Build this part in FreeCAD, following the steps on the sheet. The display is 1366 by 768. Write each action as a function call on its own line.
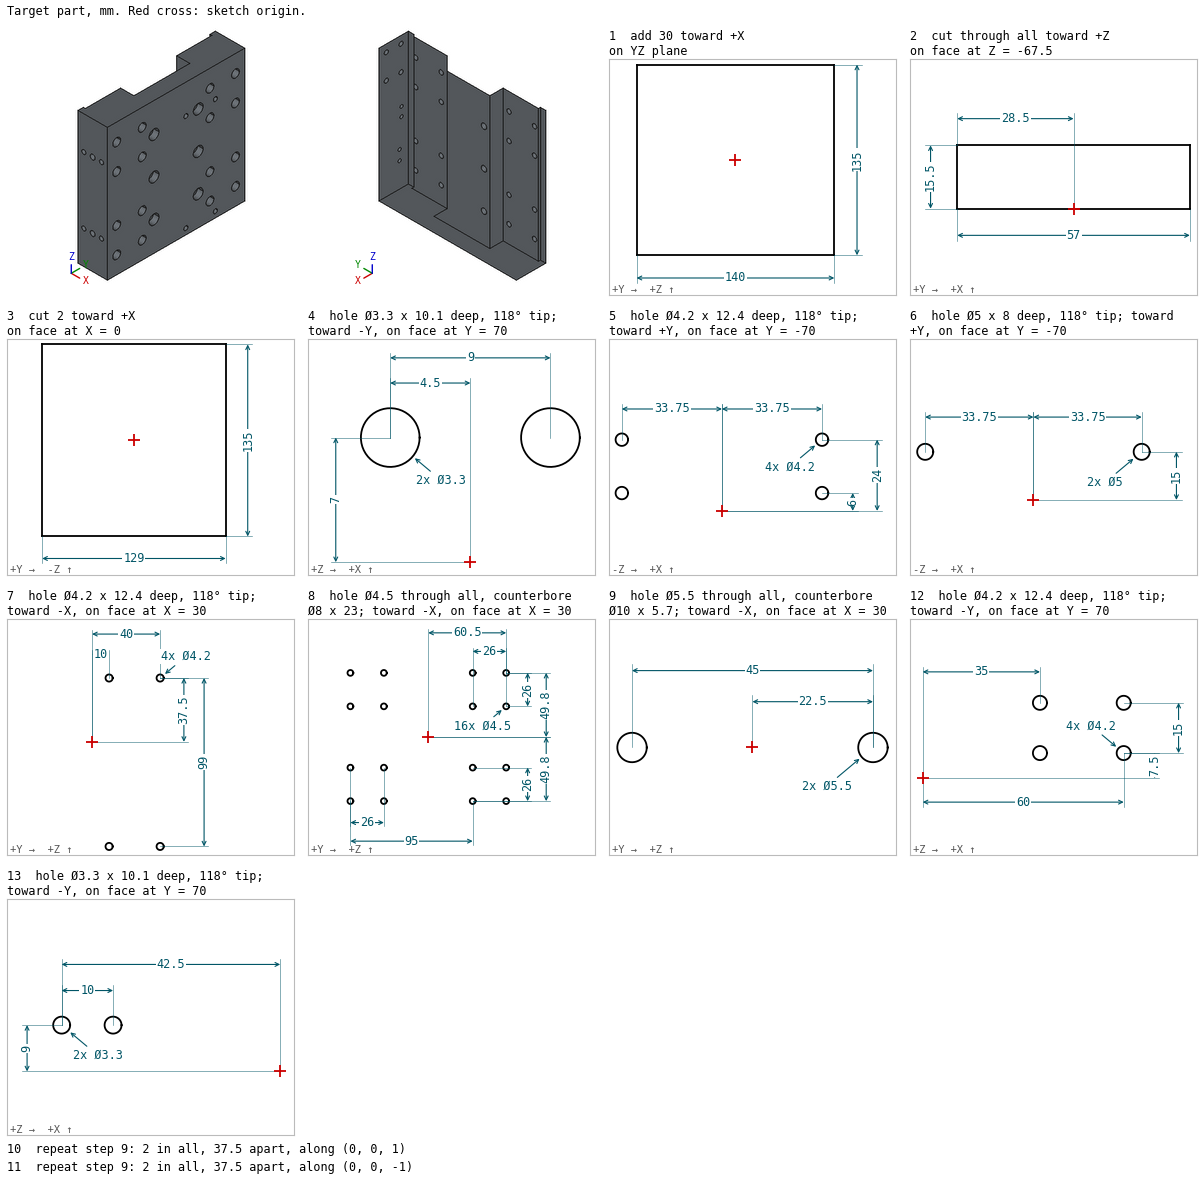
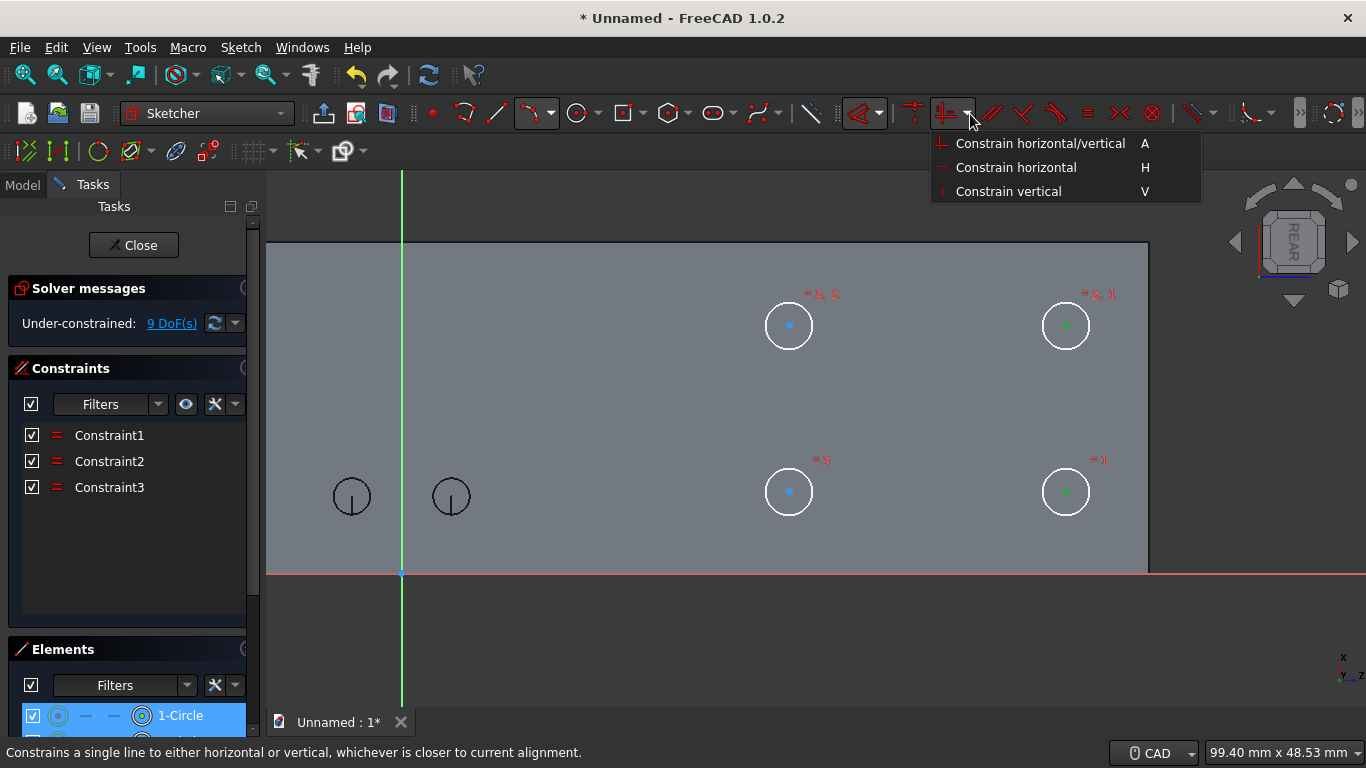
click(1066, 191)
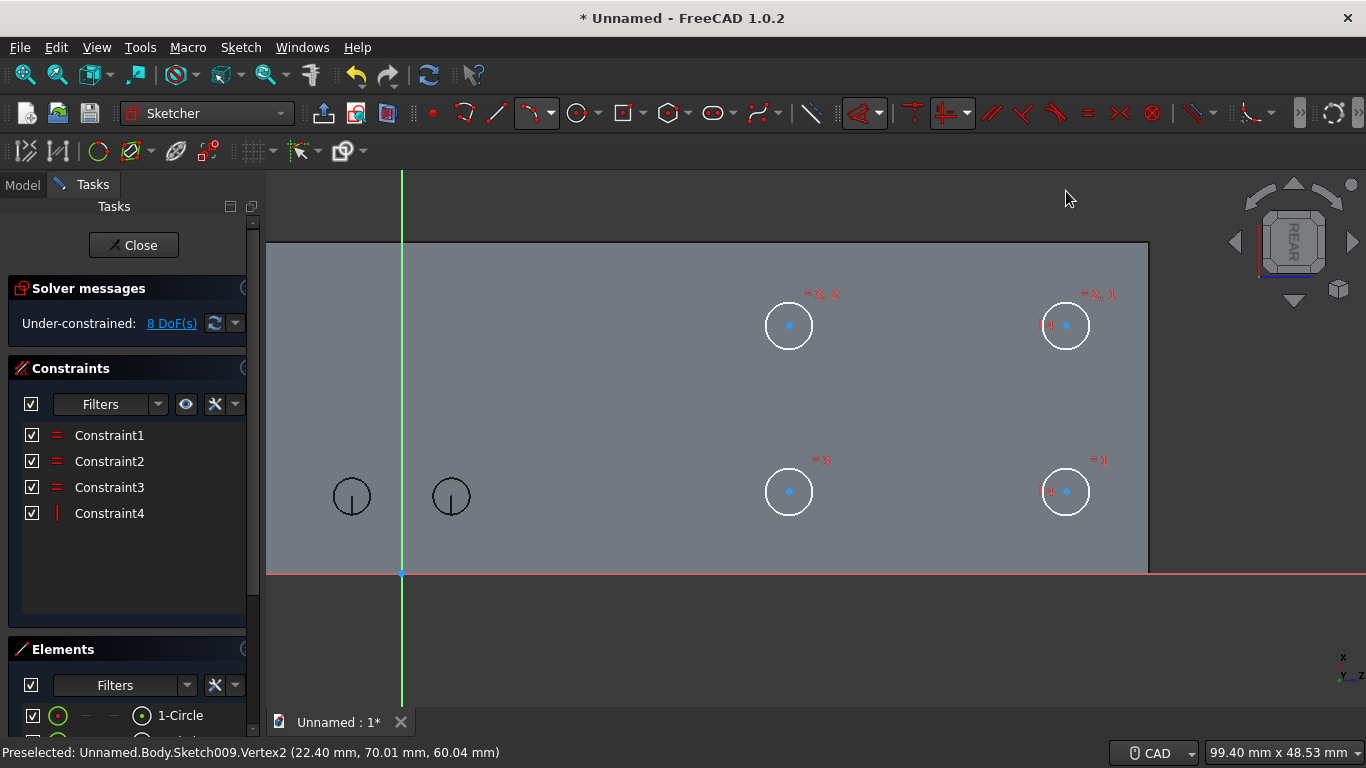
click(1066, 326)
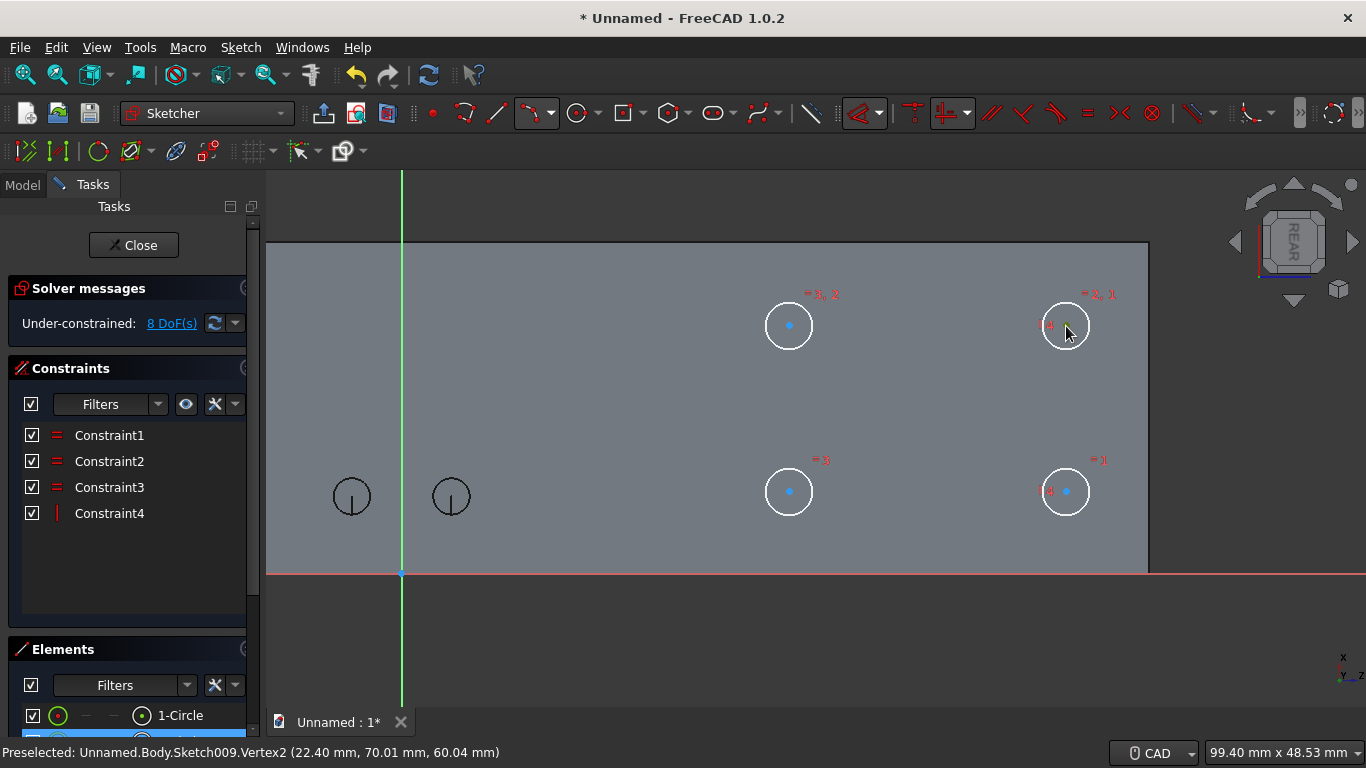
click(789, 326)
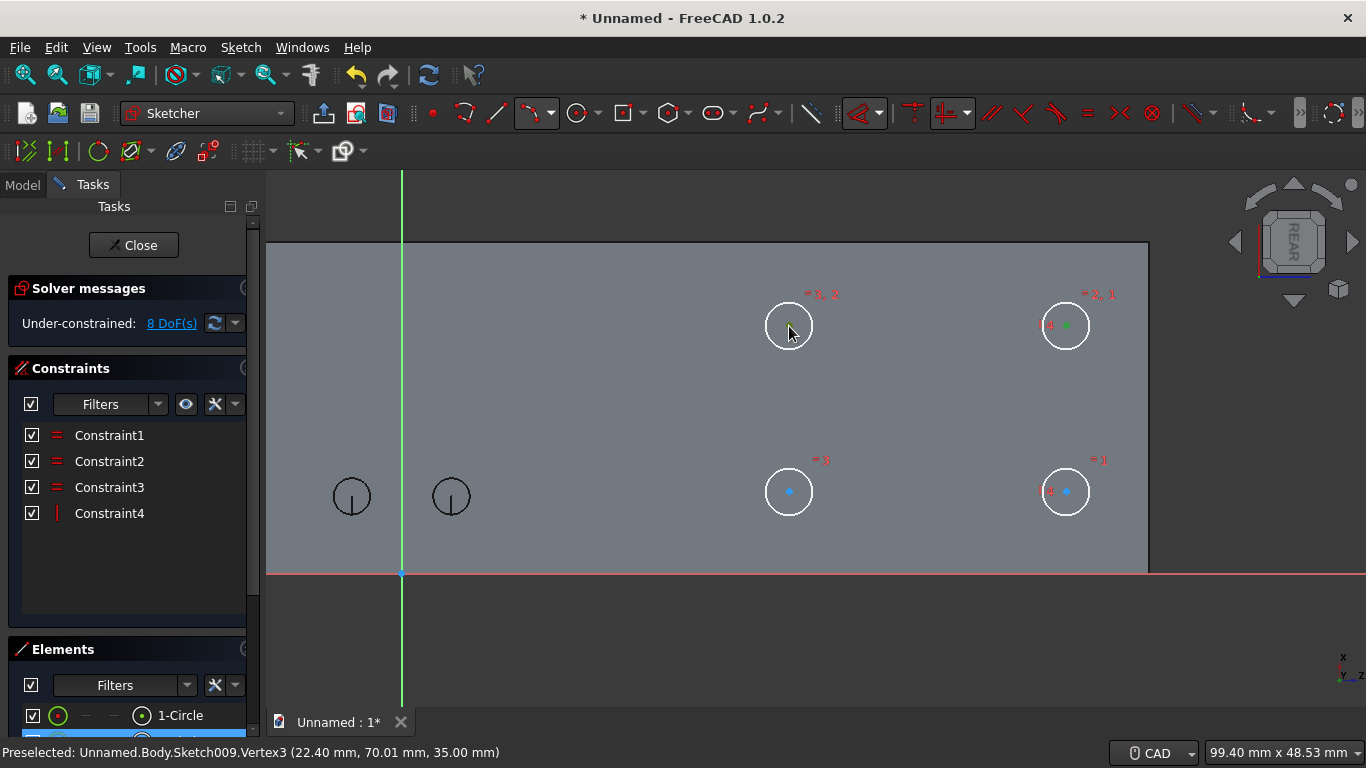
key(h)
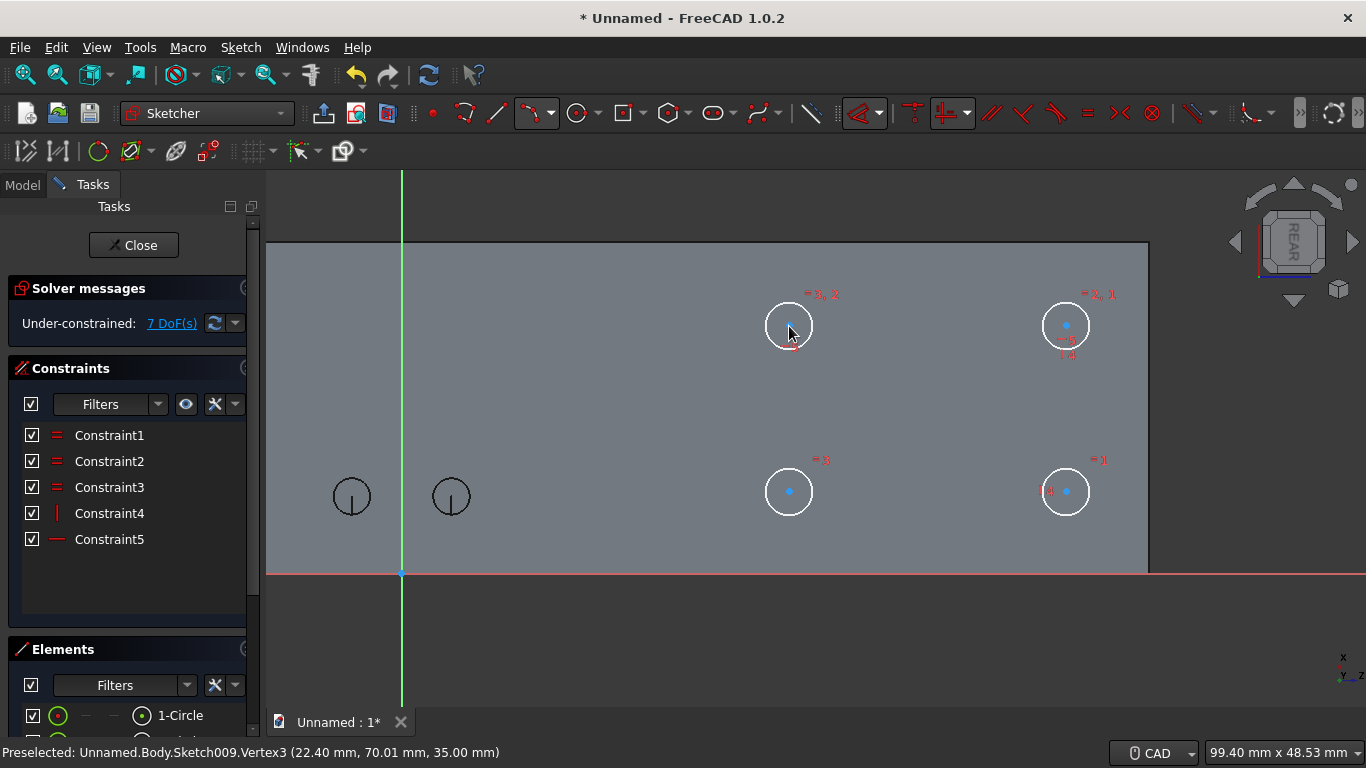
click(789, 326)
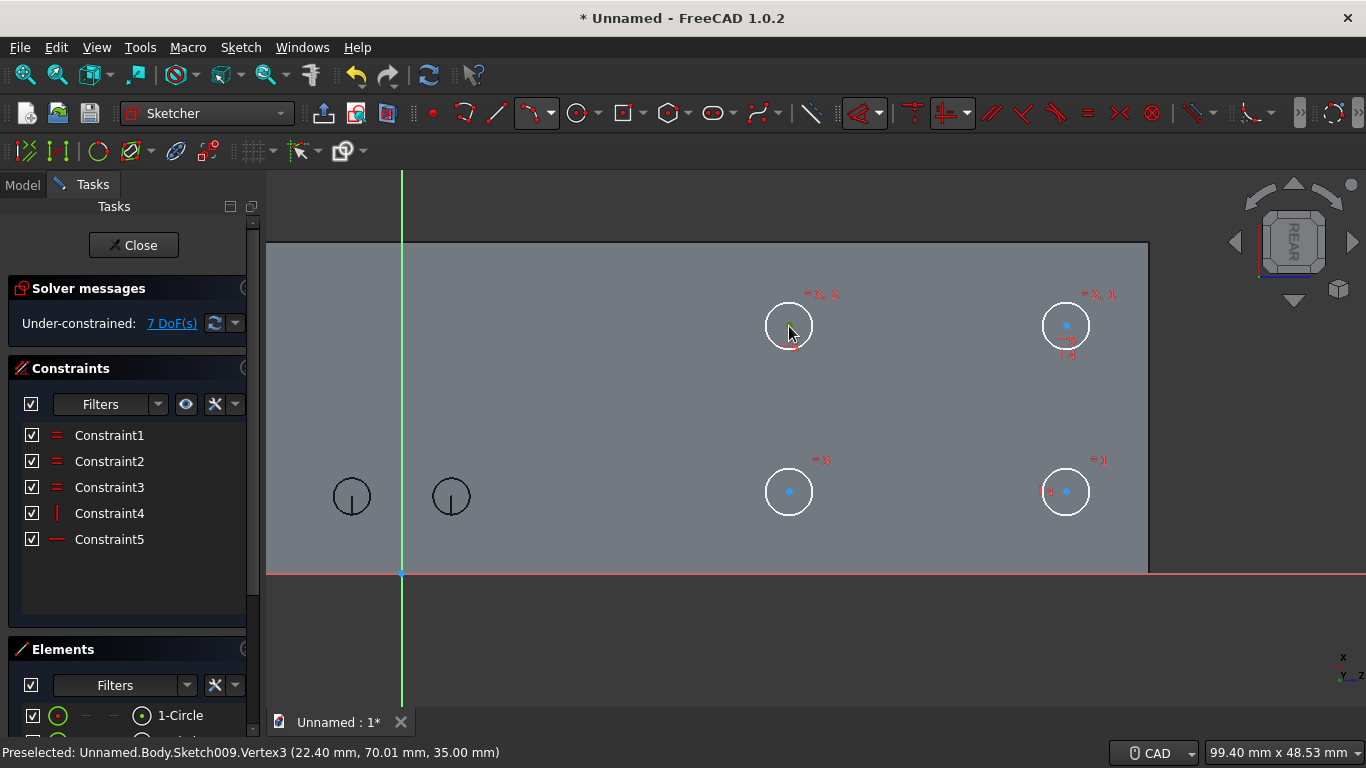
click(789, 492)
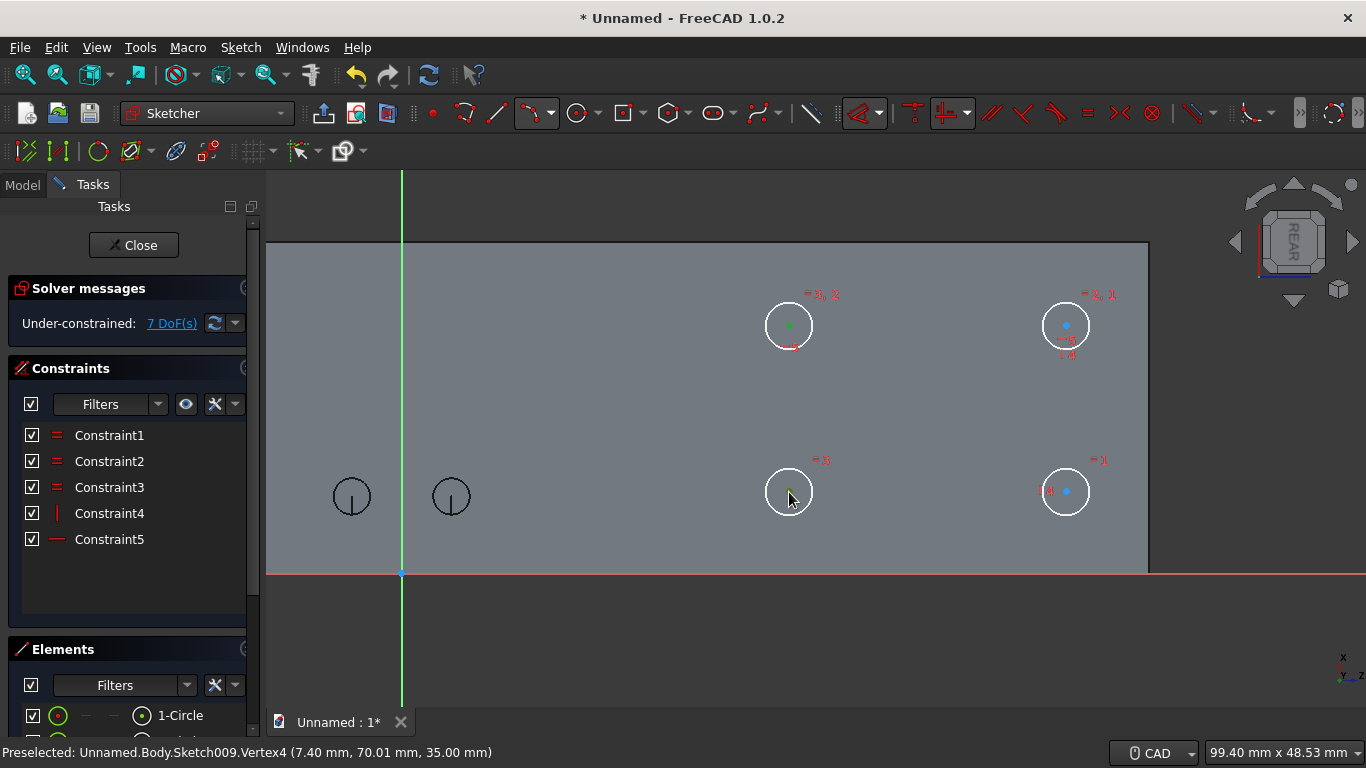
key(v)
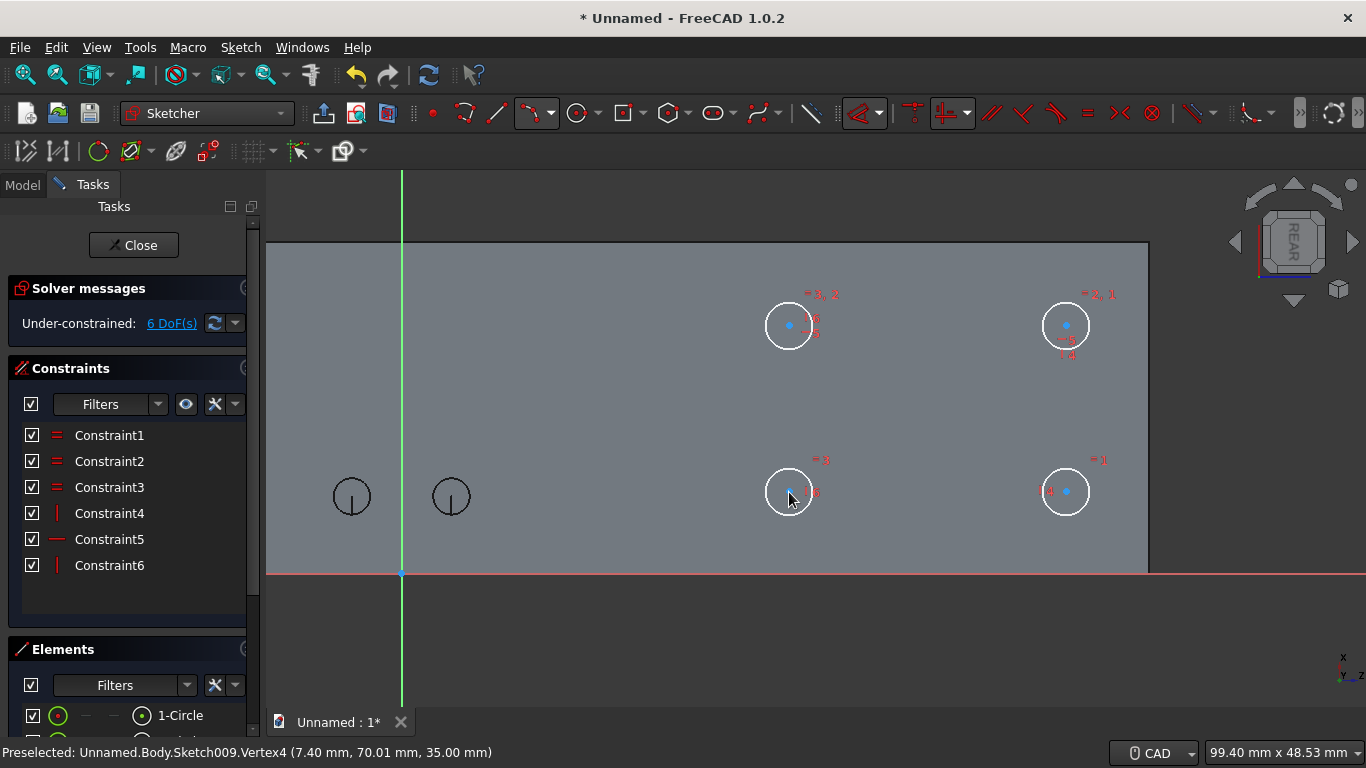
click(1066, 492)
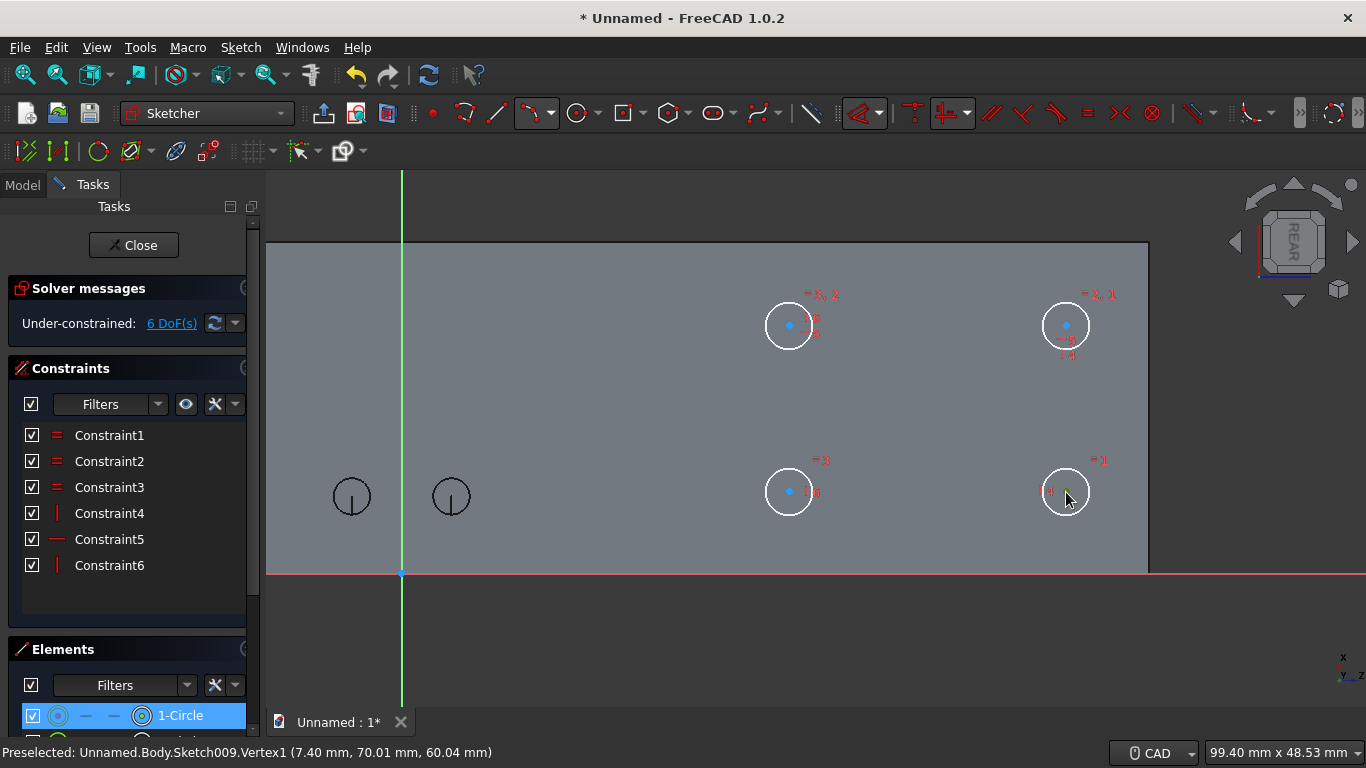
click(789, 492)